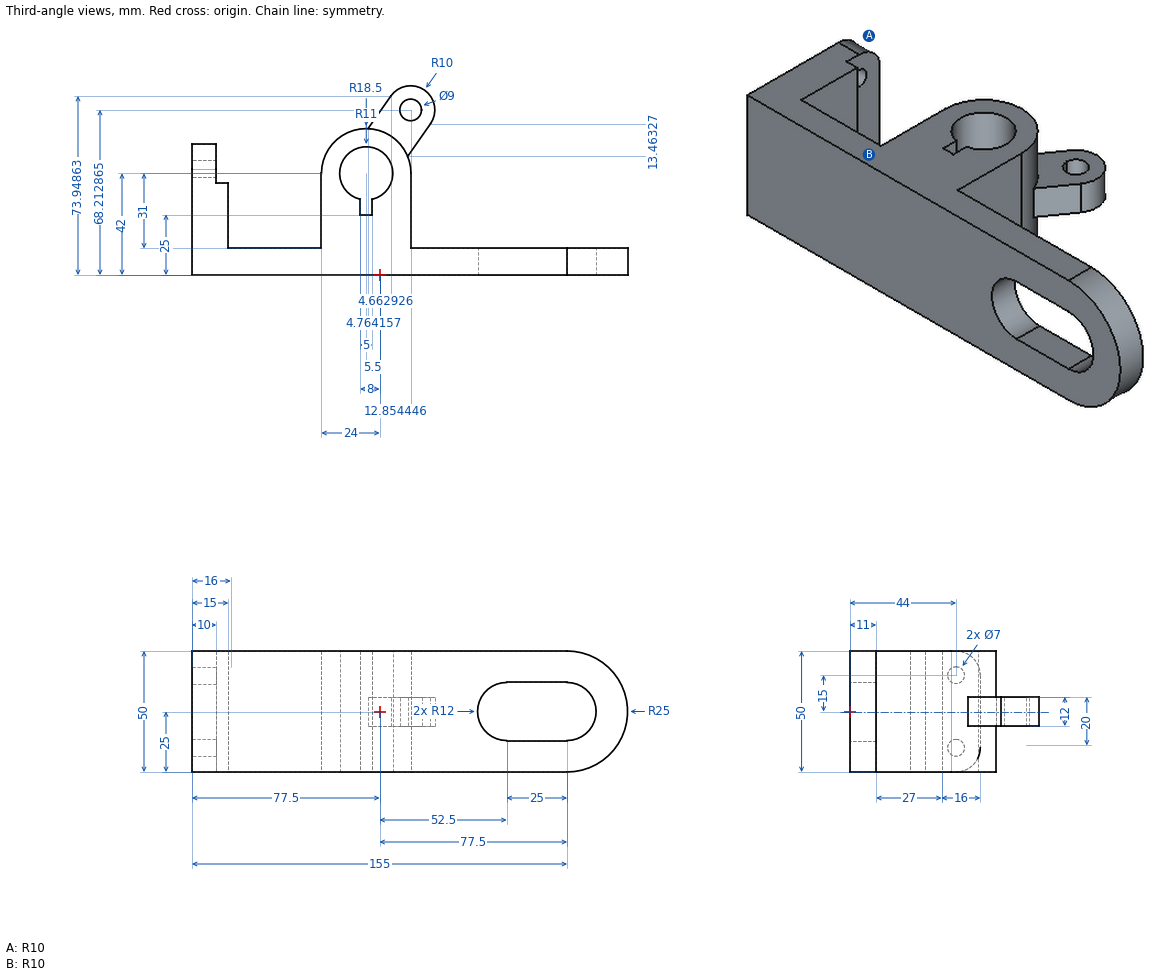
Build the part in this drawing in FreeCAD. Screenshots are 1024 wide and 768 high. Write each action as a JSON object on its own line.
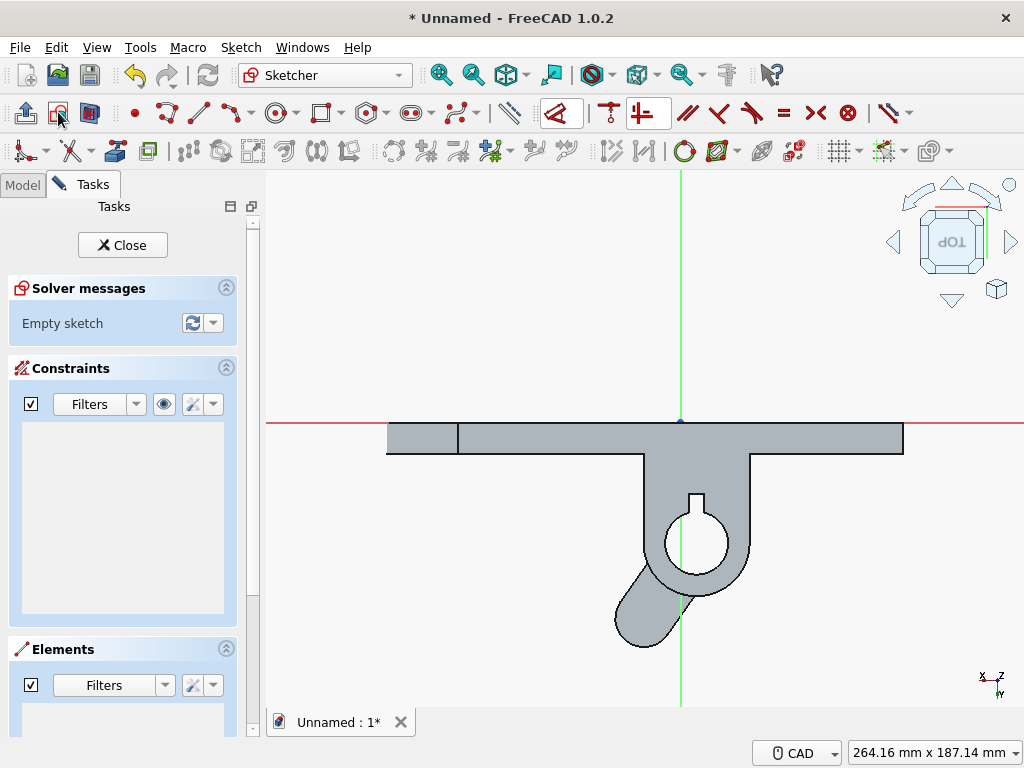
{"action": "scroll", "coordinate": [649, 633], "scroll_direction": "up", "scroll_amount": 13}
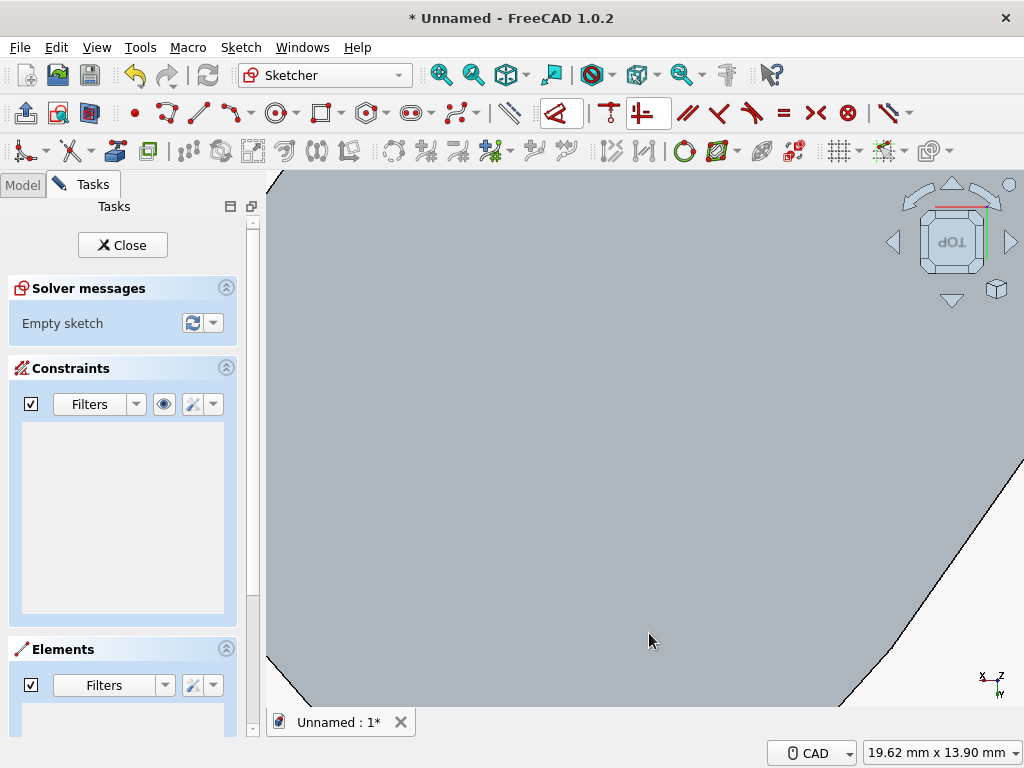
{"action": "left_click", "coordinate": [276, 114]}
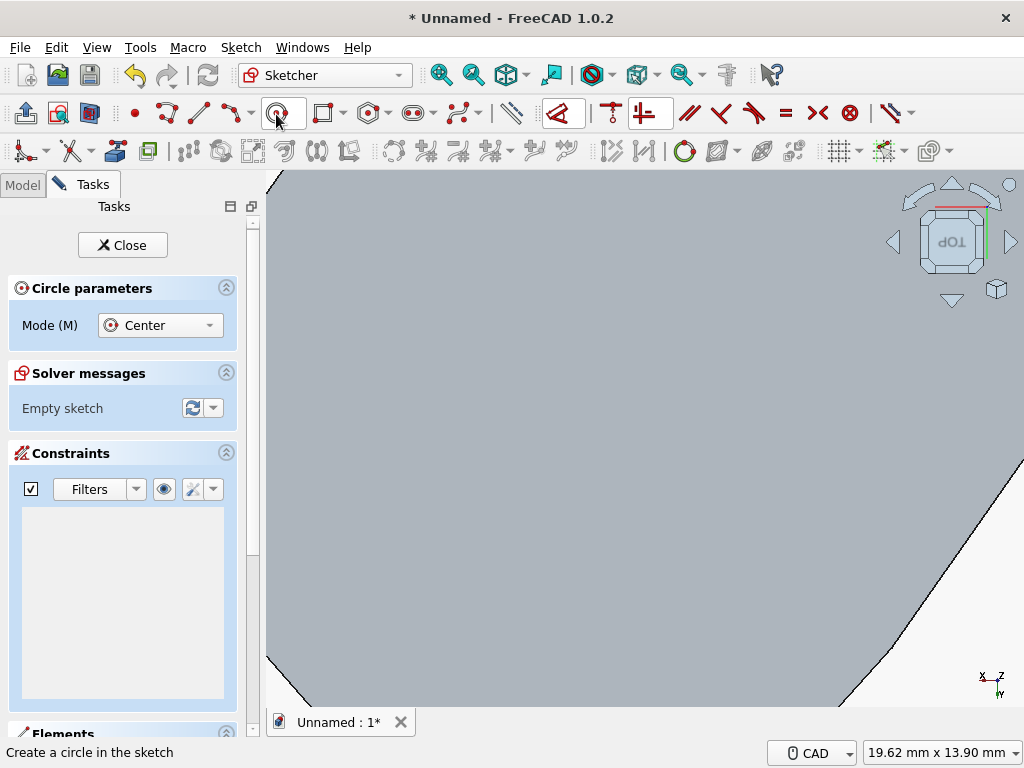
{"action": "left_click", "coordinate": [575, 426]}
{"action": "left_click", "coordinate": [698, 303]}
{"action": "key", "text": "Escape"}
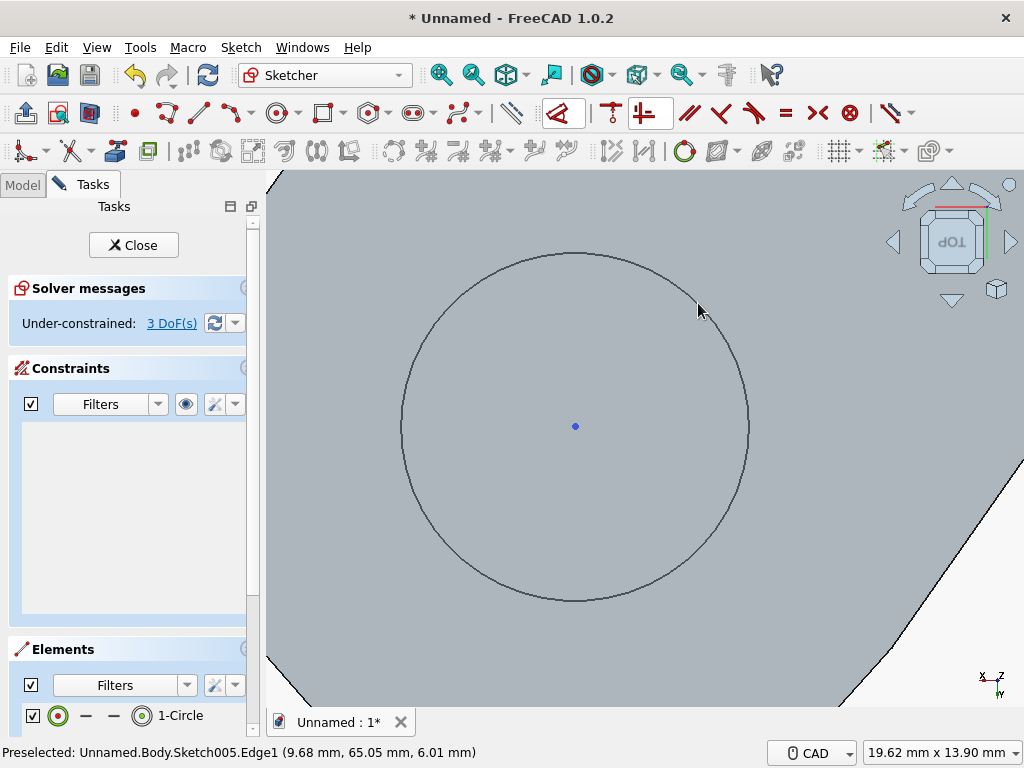
{"action": "left_click", "coordinate": [698, 304]}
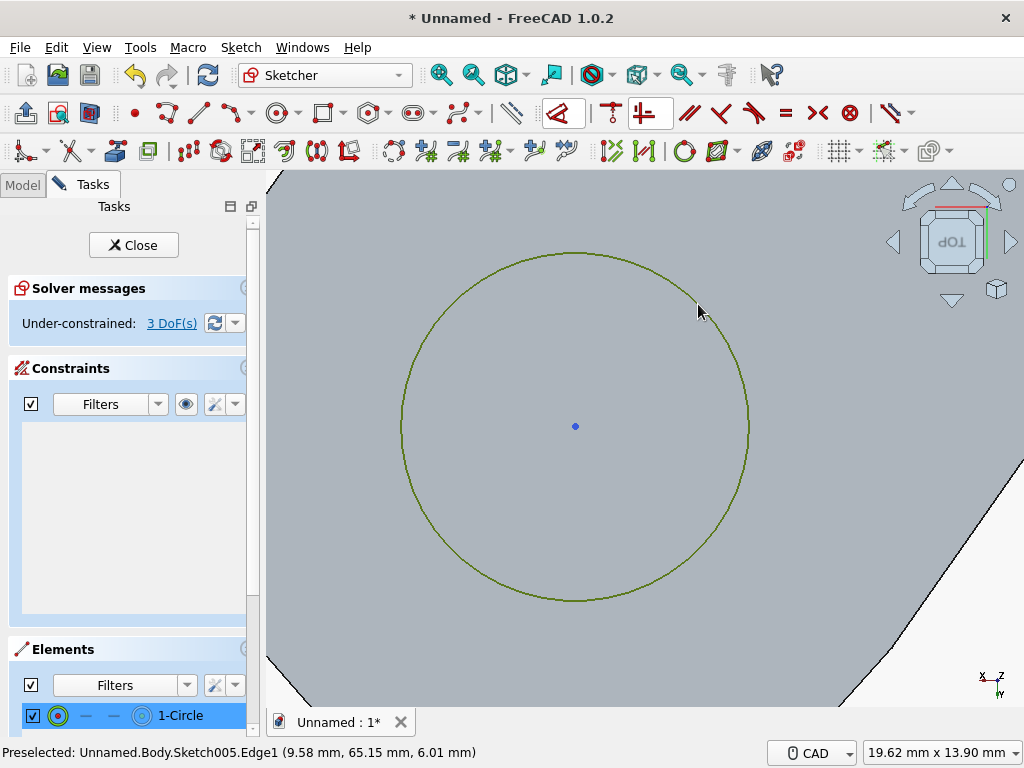
{"action": "left_click", "coordinate": [580, 114]}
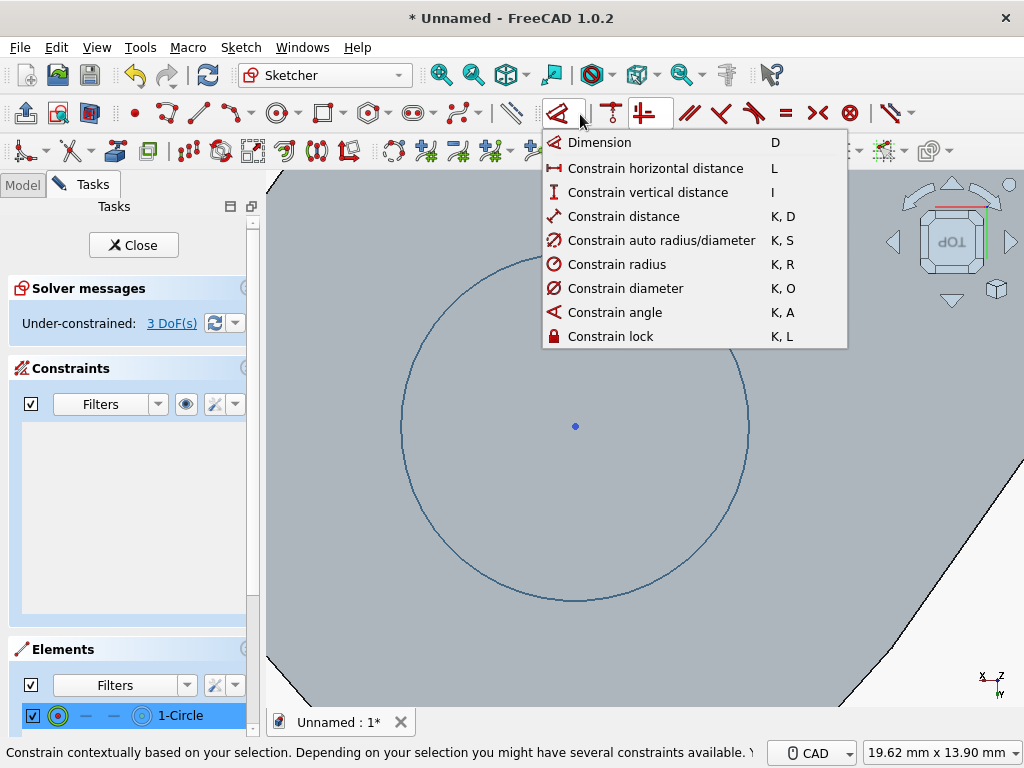
{"action": "left_click", "coordinate": [695, 288]}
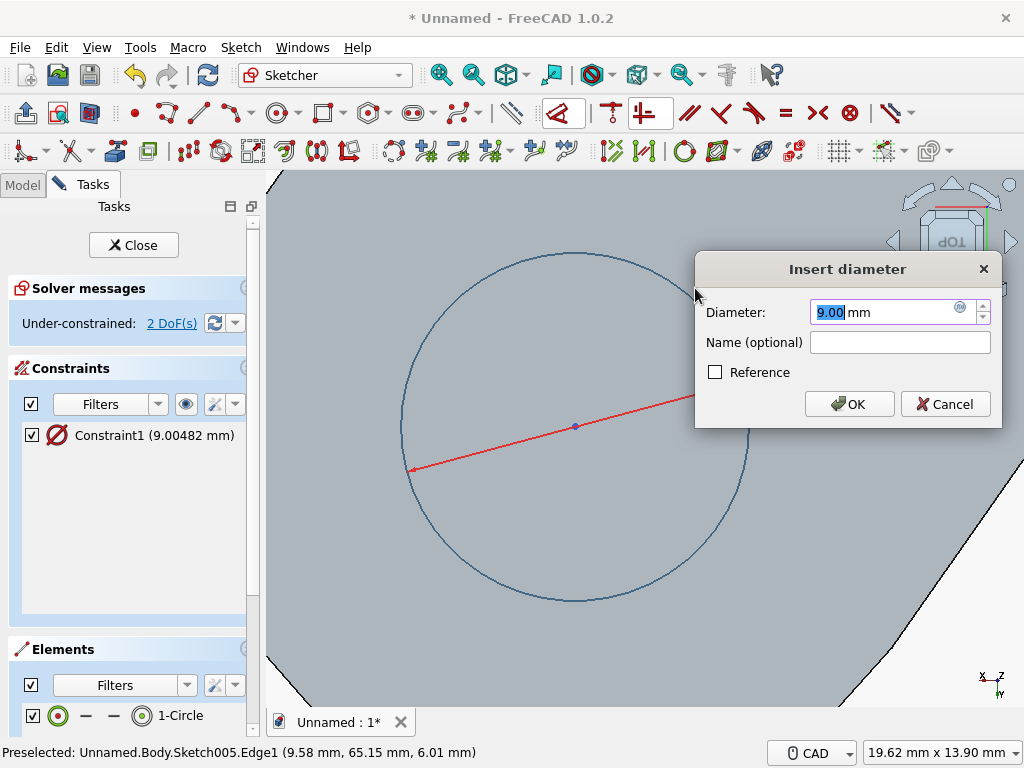
{"action": "type", "text": "9"}
{"action": "key", "text": "Return"}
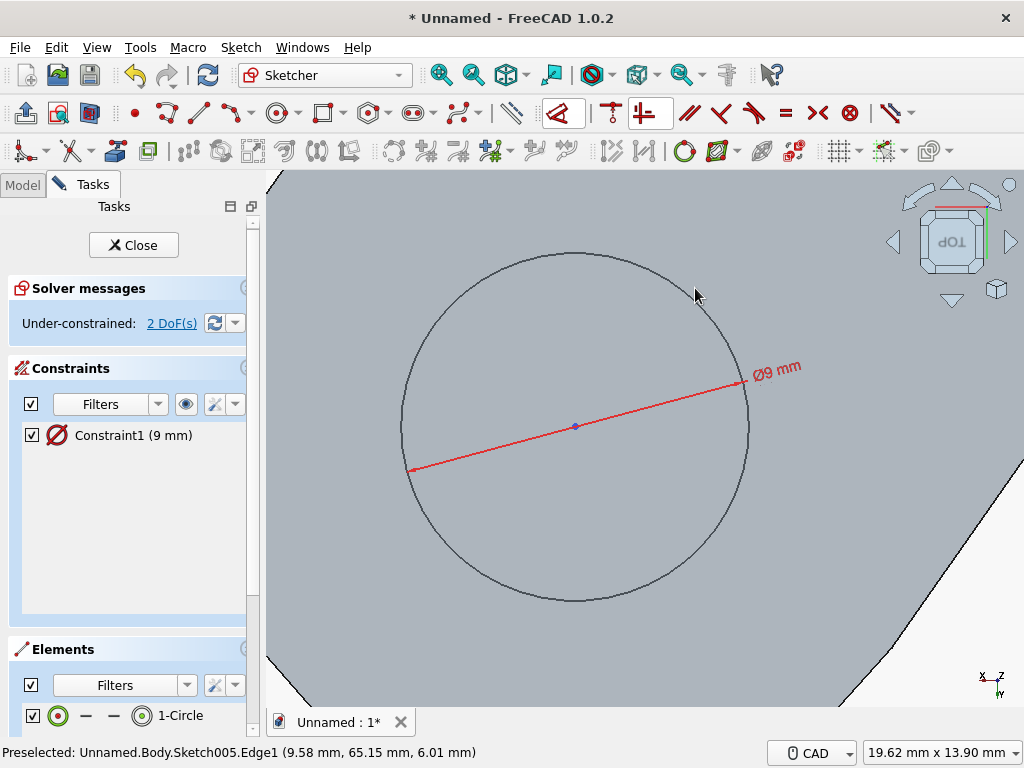
{"action": "left_click", "coordinate": [575, 427]}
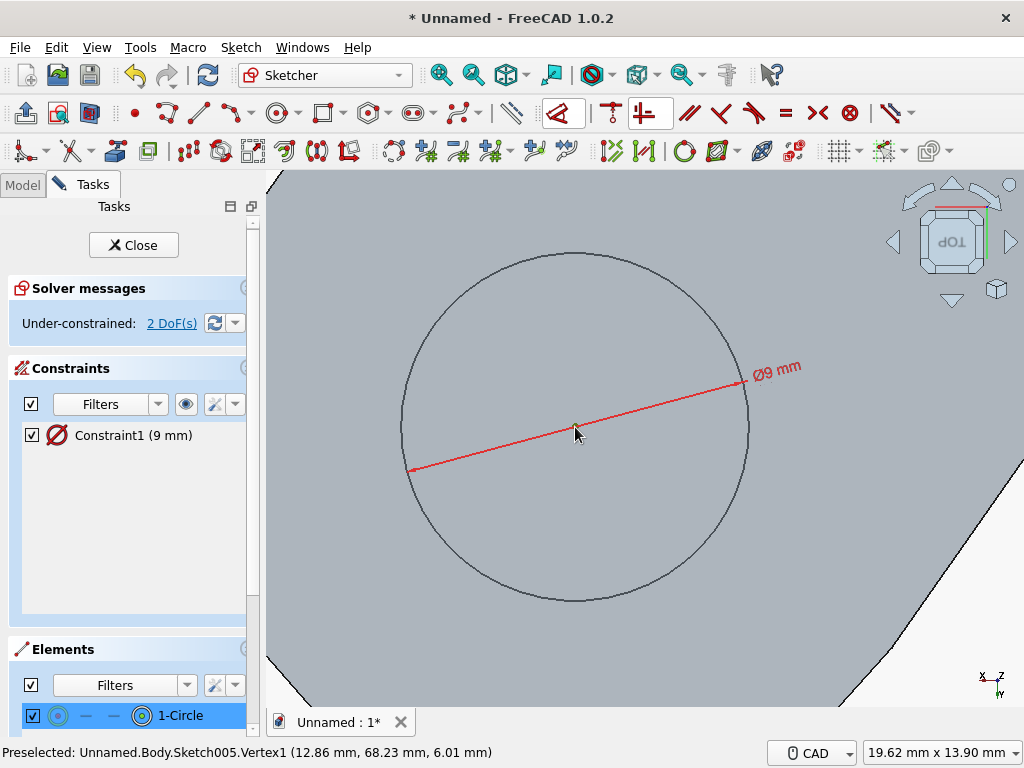
{"action": "left_click", "coordinate": [580, 114]}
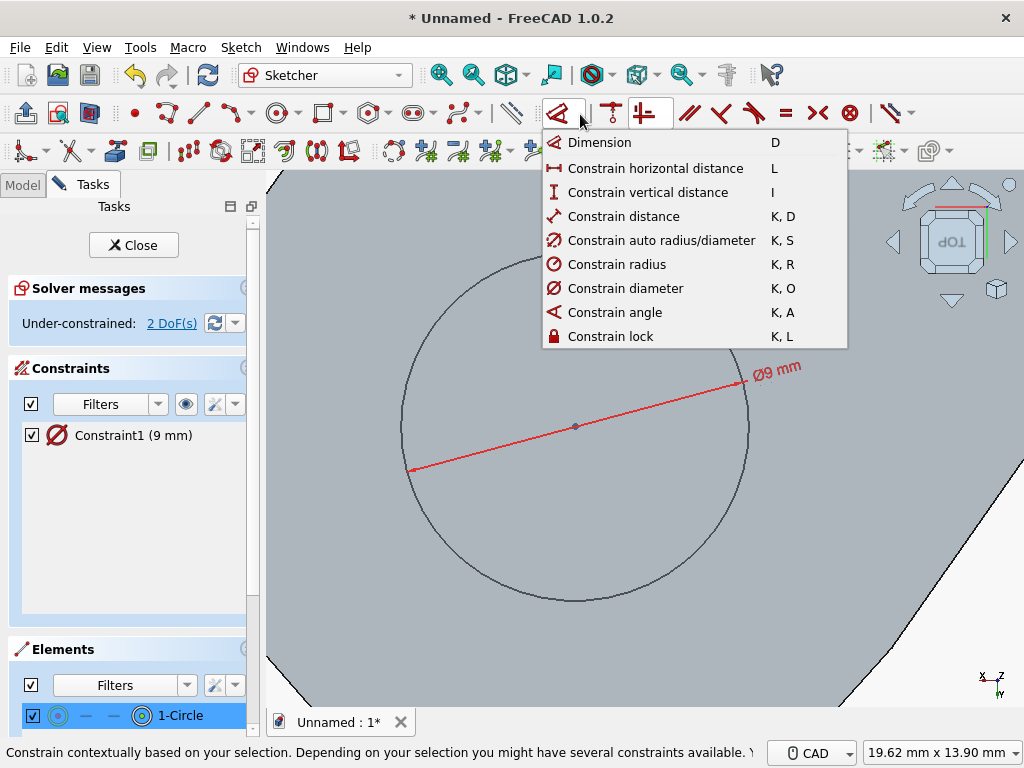
{"action": "left_click", "coordinate": [695, 168]}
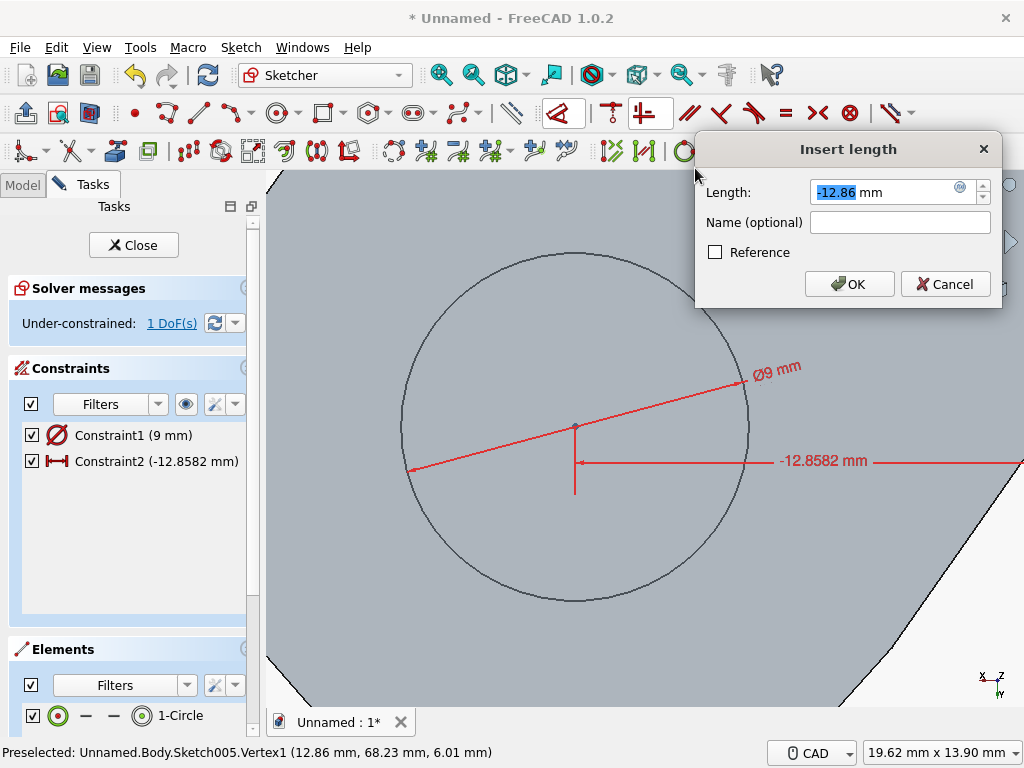
{"action": "type", "text": "-12.854446"}
{"action": "key", "text": "Return"}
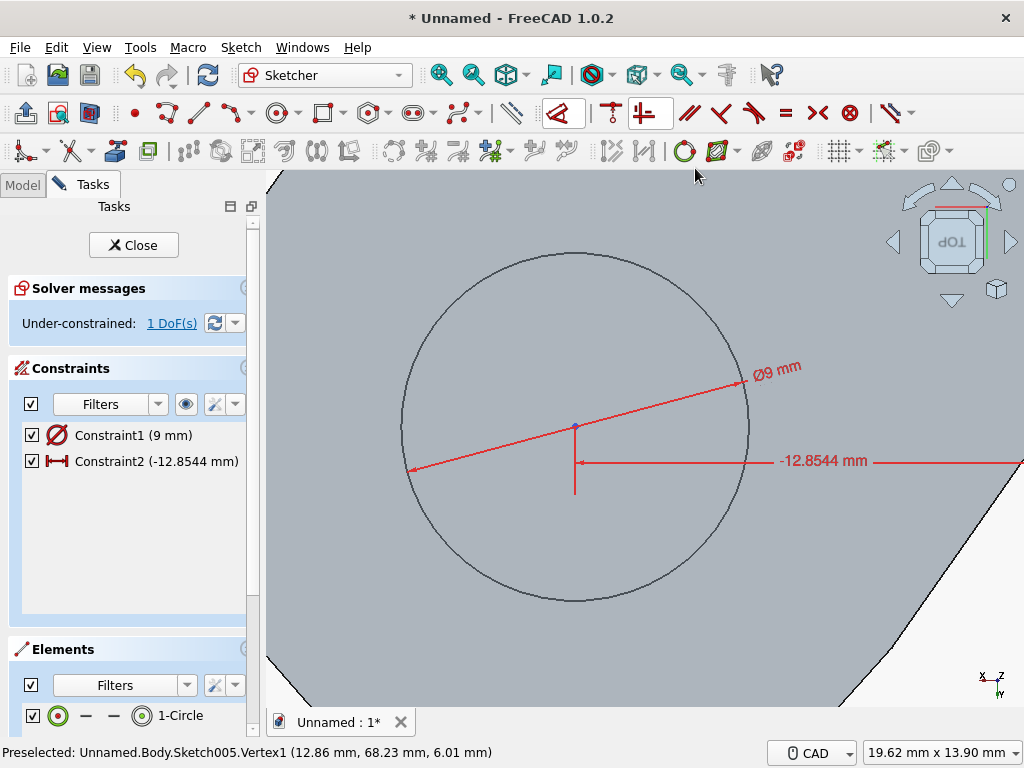
{"action": "left_click", "coordinate": [575, 427]}